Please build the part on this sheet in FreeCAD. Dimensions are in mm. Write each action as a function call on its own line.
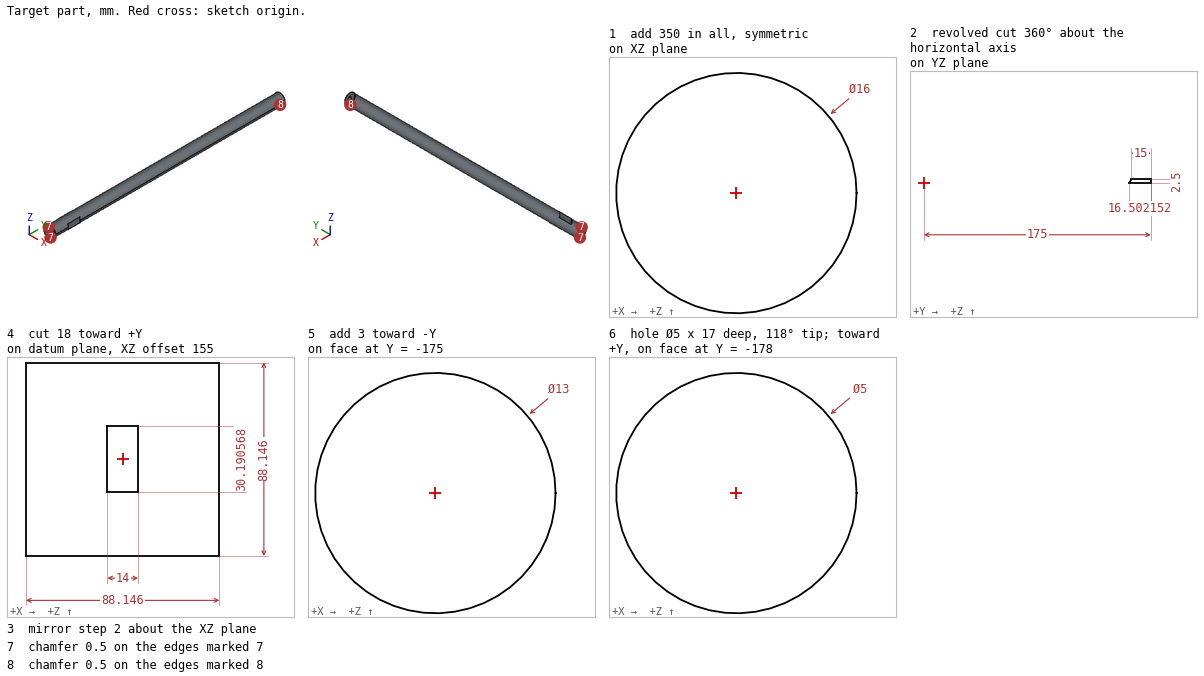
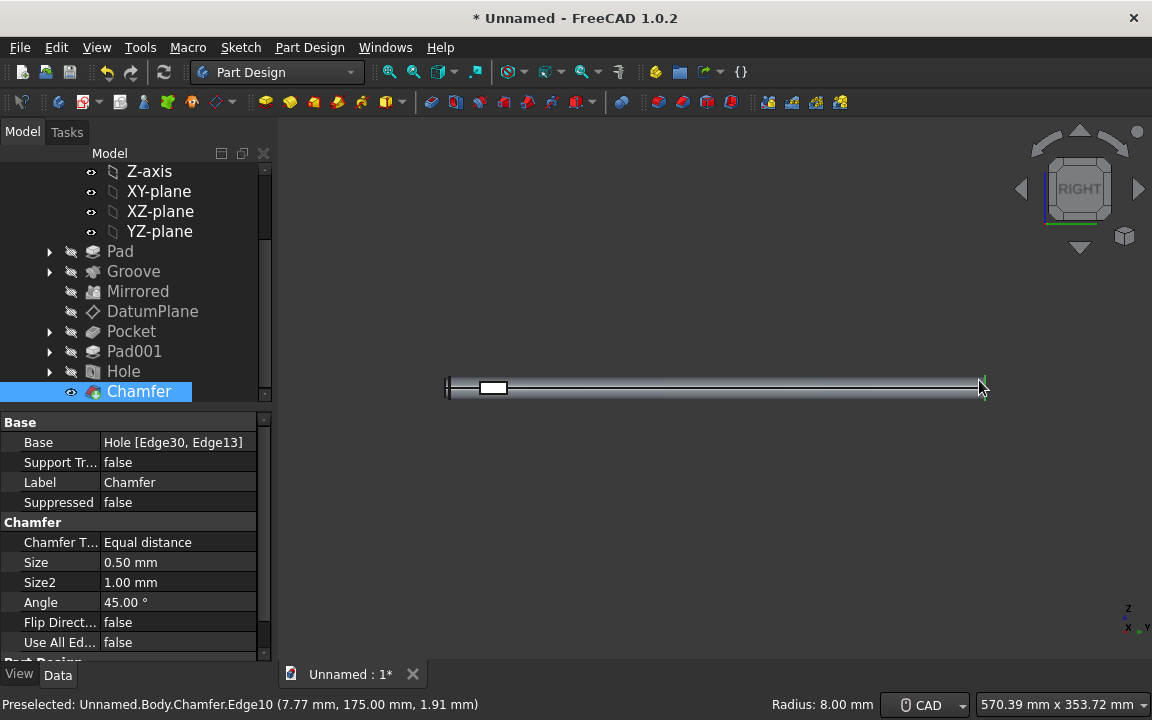
click(684, 102)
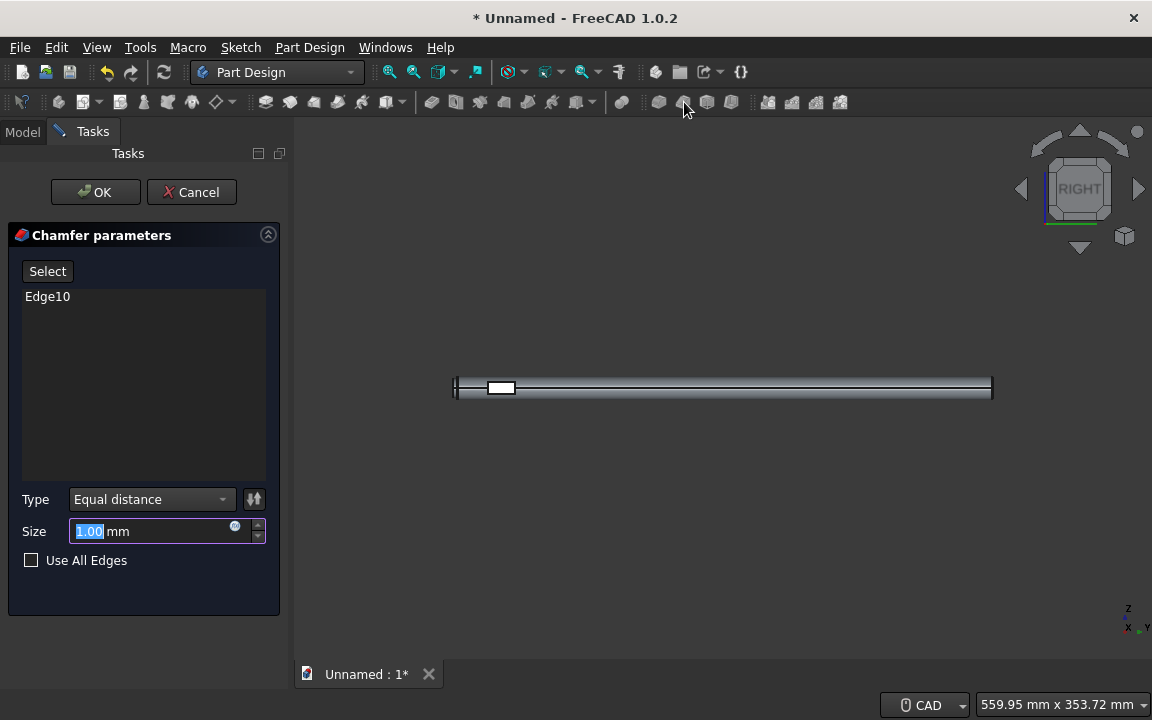
text(0.5)
key(Tab)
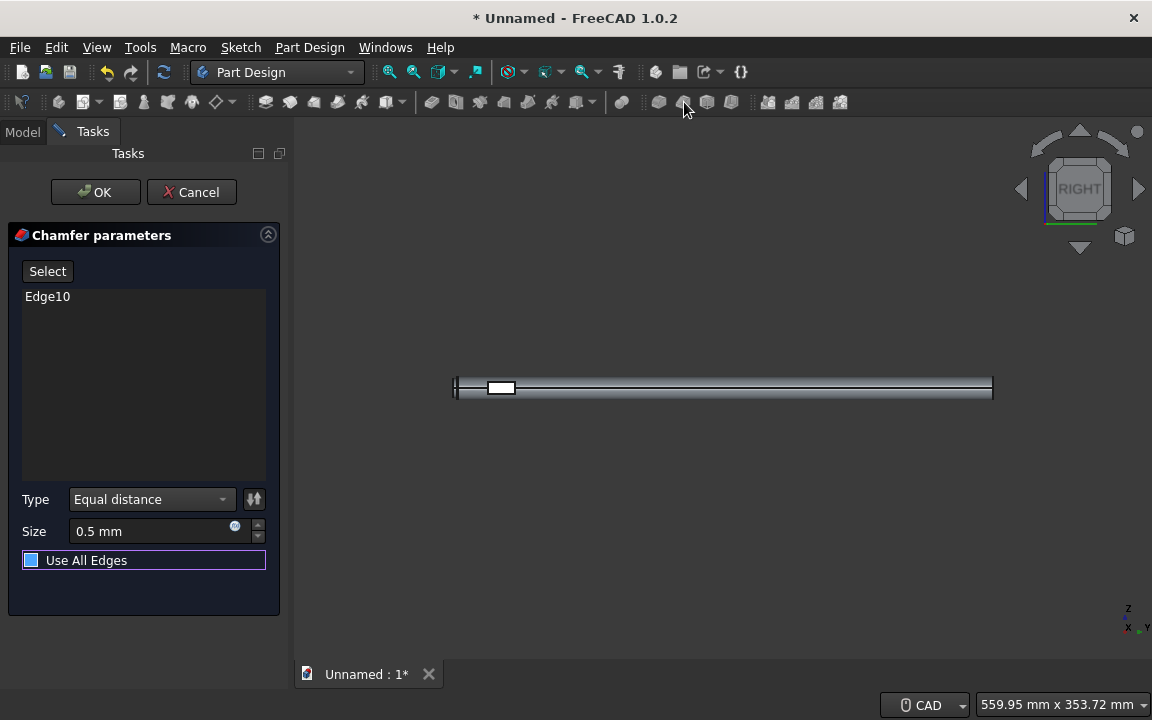
click(96, 192)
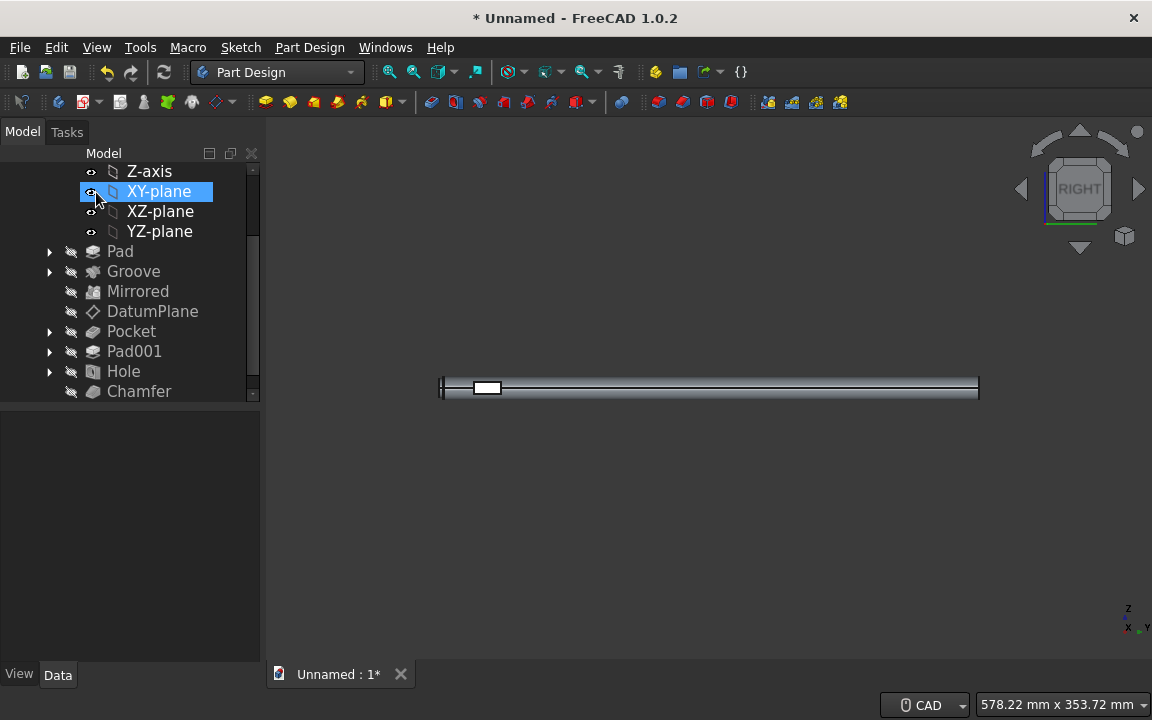
key(0)